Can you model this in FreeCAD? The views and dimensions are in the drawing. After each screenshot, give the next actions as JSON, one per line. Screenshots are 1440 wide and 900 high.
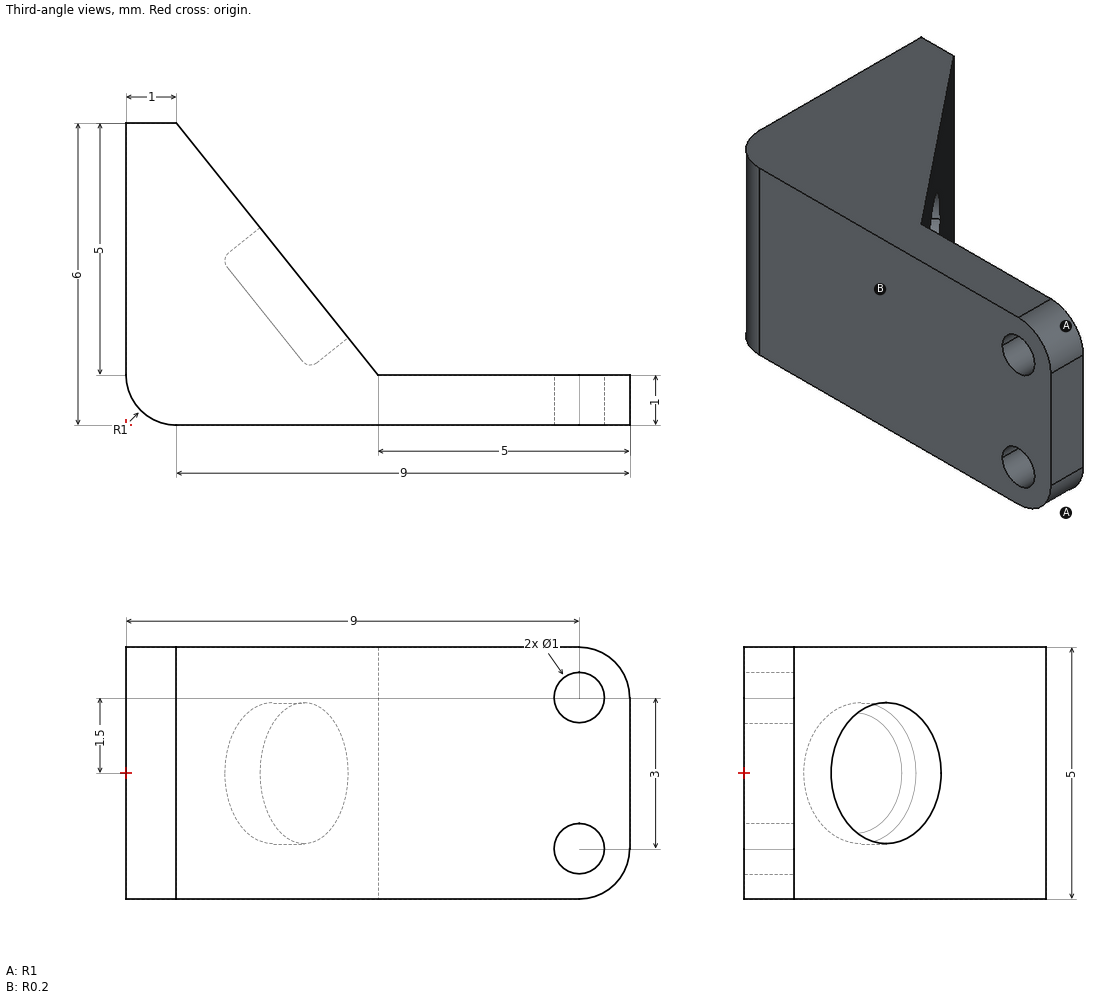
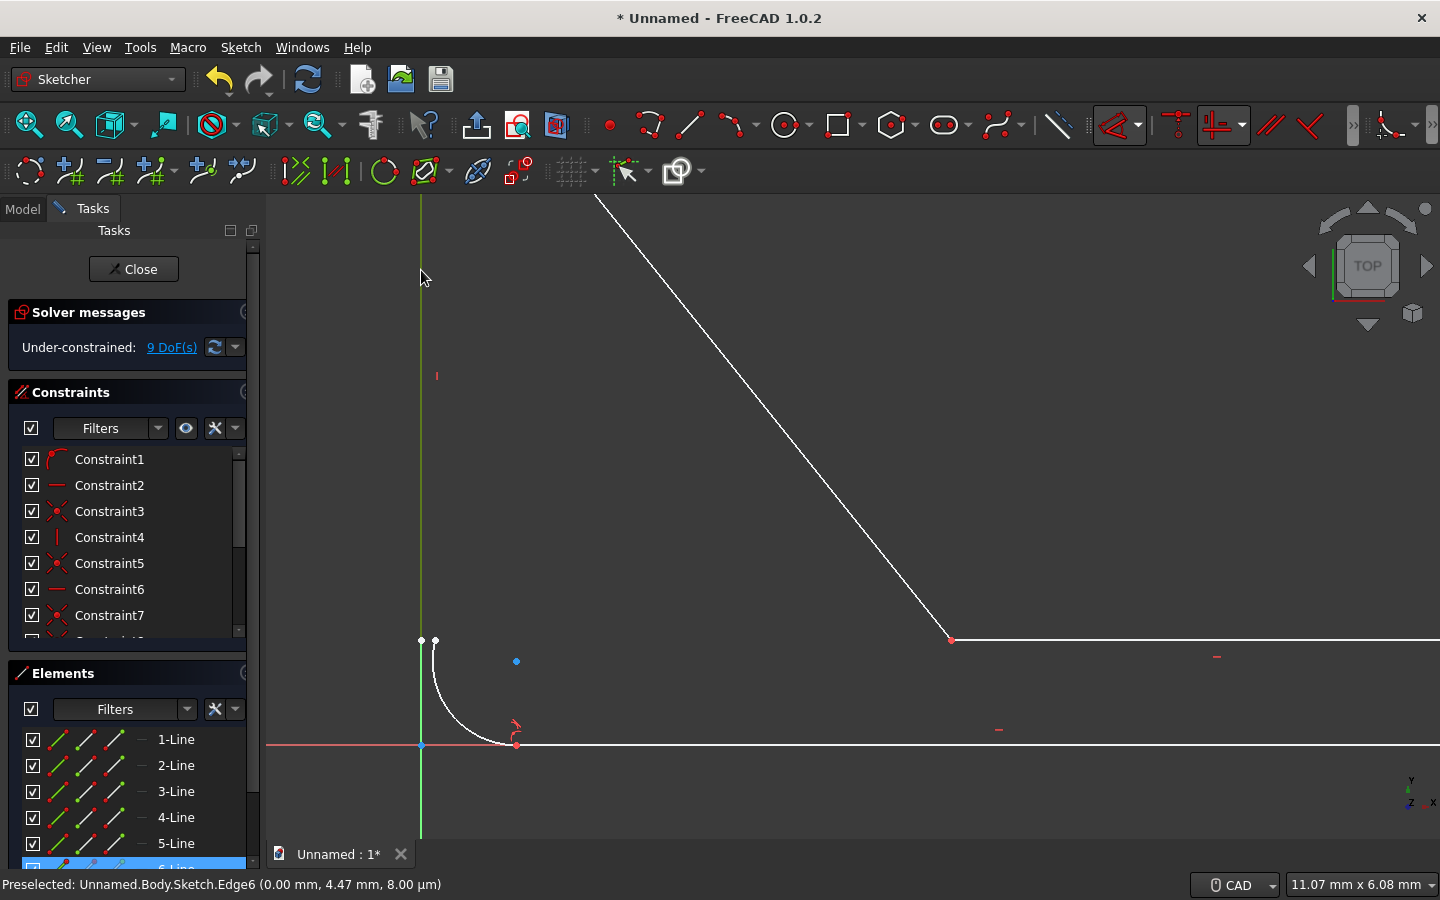
{"action": "left_click", "coordinate": [436, 686]}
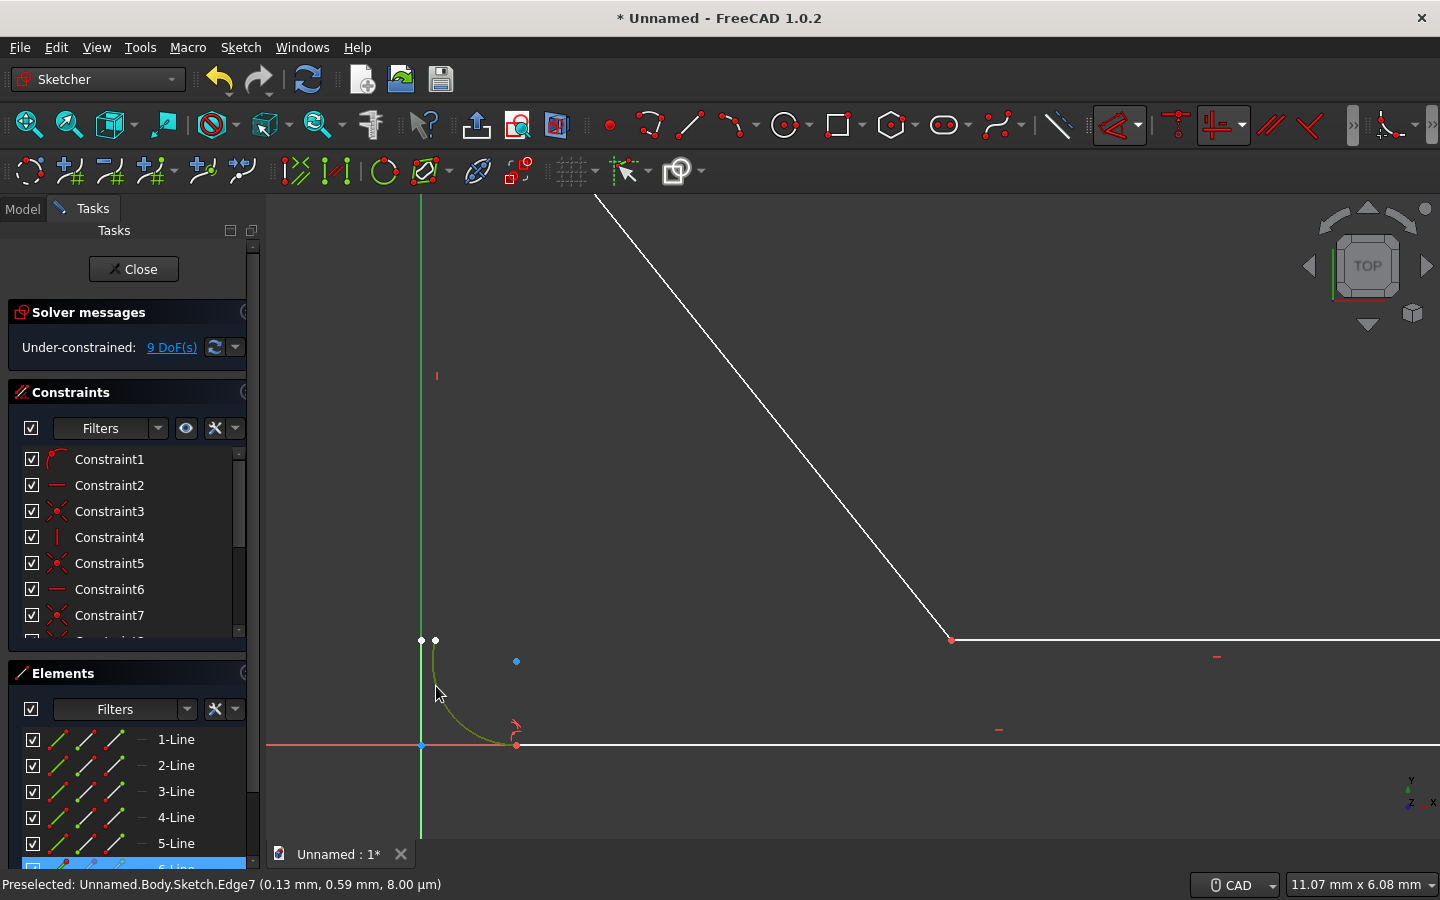
{"action": "key", "text": "t"}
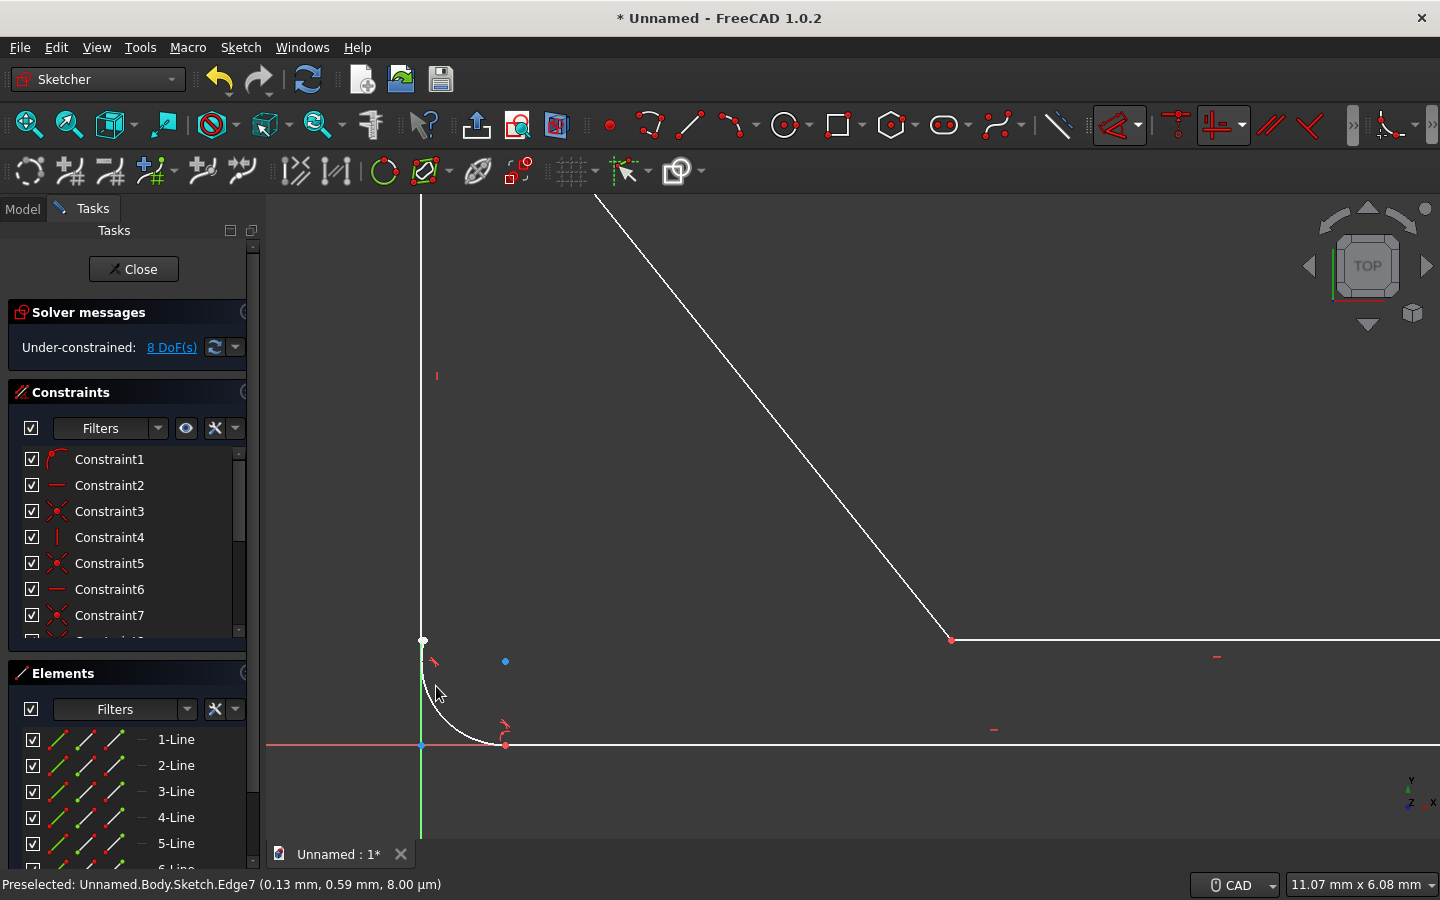
{"action": "left_click", "coordinate": [1114, 126]}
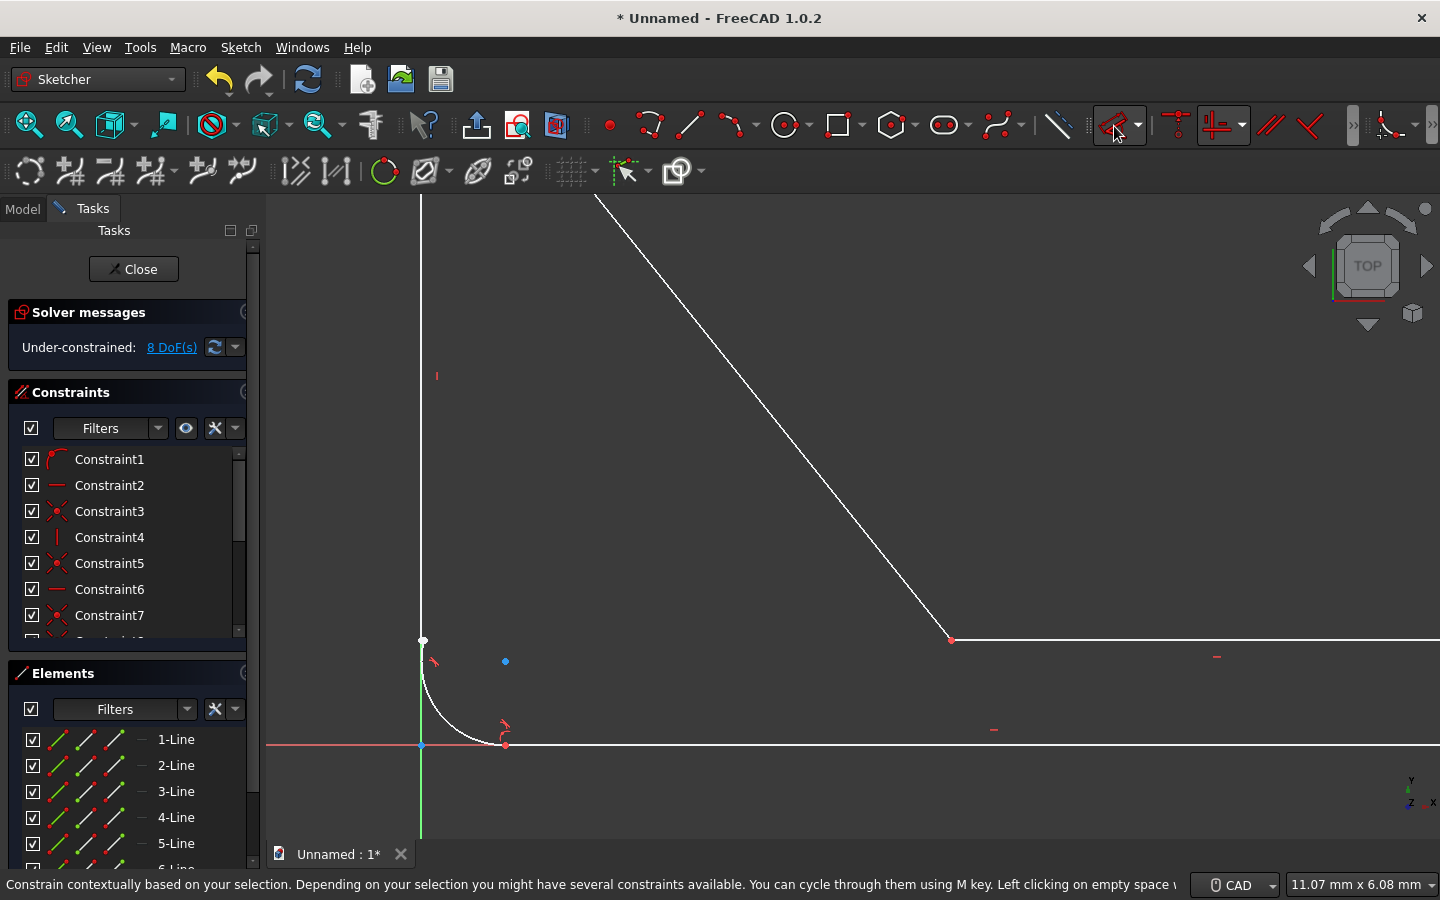
{"action": "left_click", "coordinate": [425, 686]}
{"action": "left_click", "coordinate": [394, 695]}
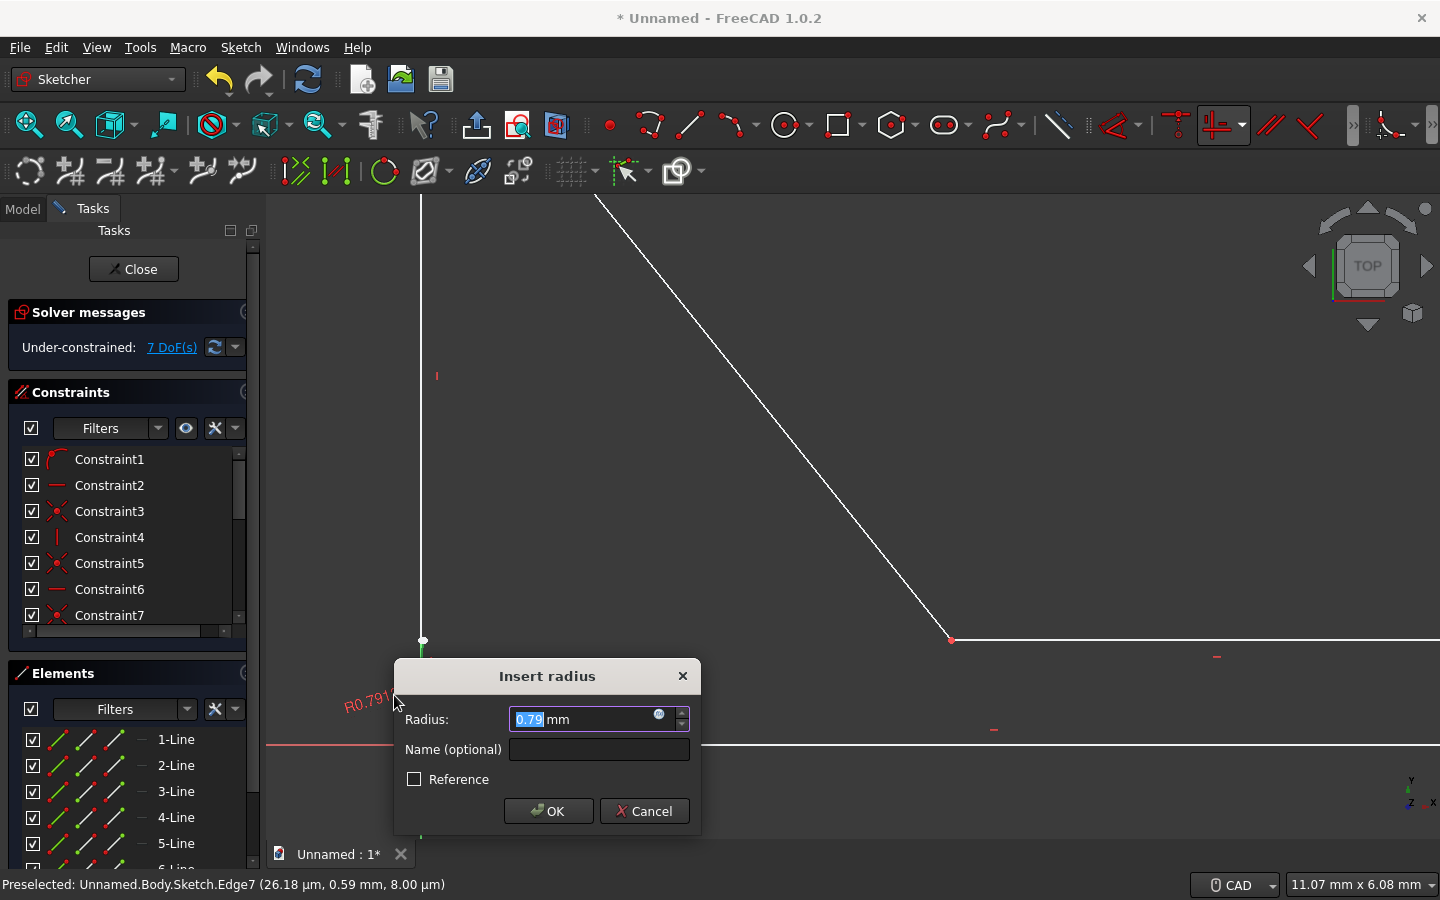
{"action": "type", "text": "1"}
{"action": "key", "text": "Return"}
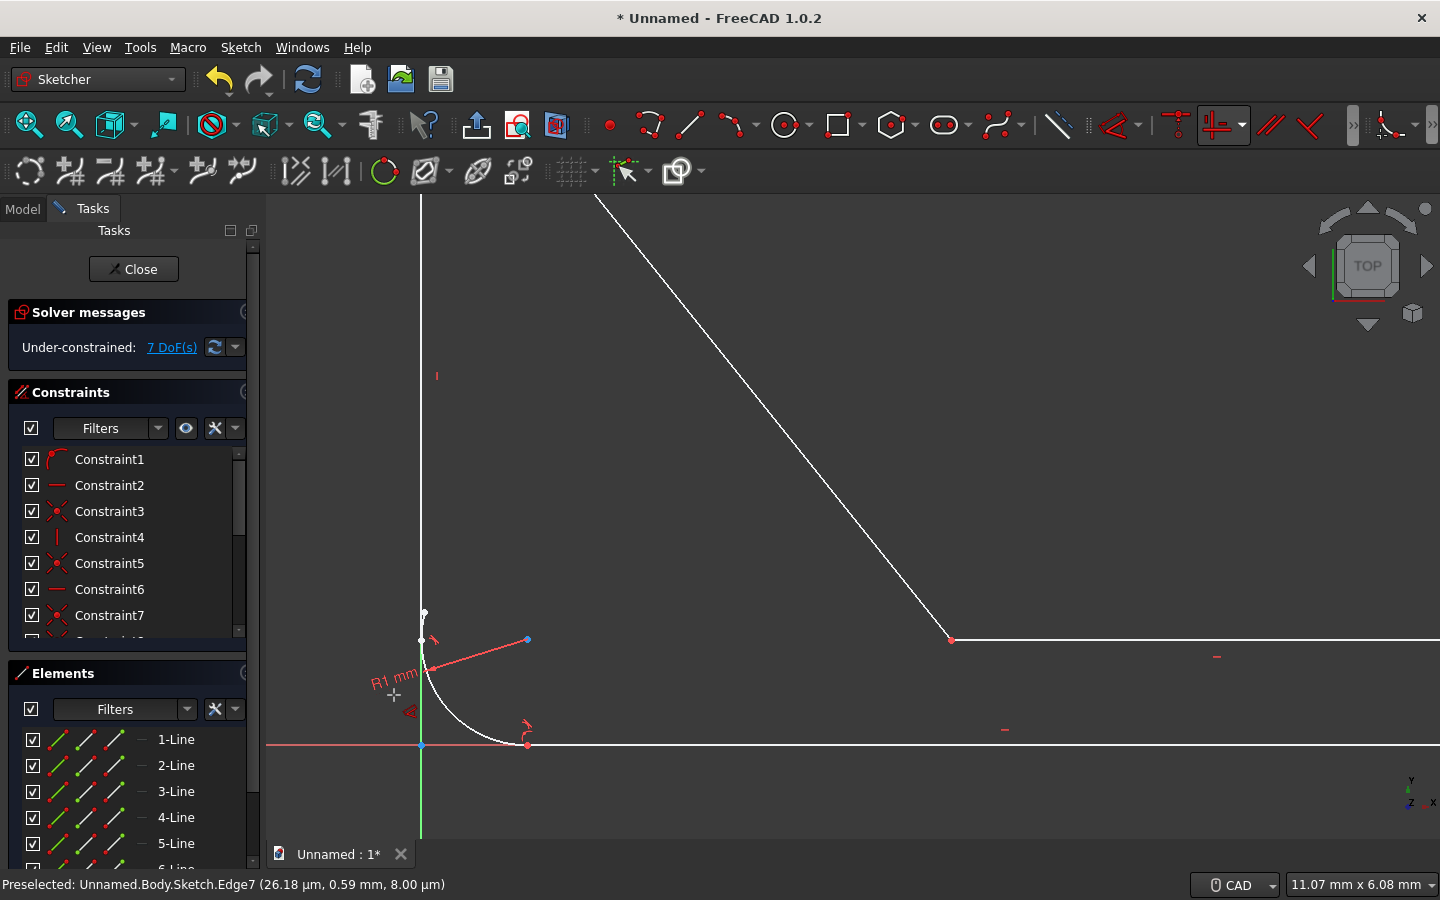
{"action": "left_click", "coordinate": [814, 745]}
{"action": "left_click", "coordinate": [901, 779]}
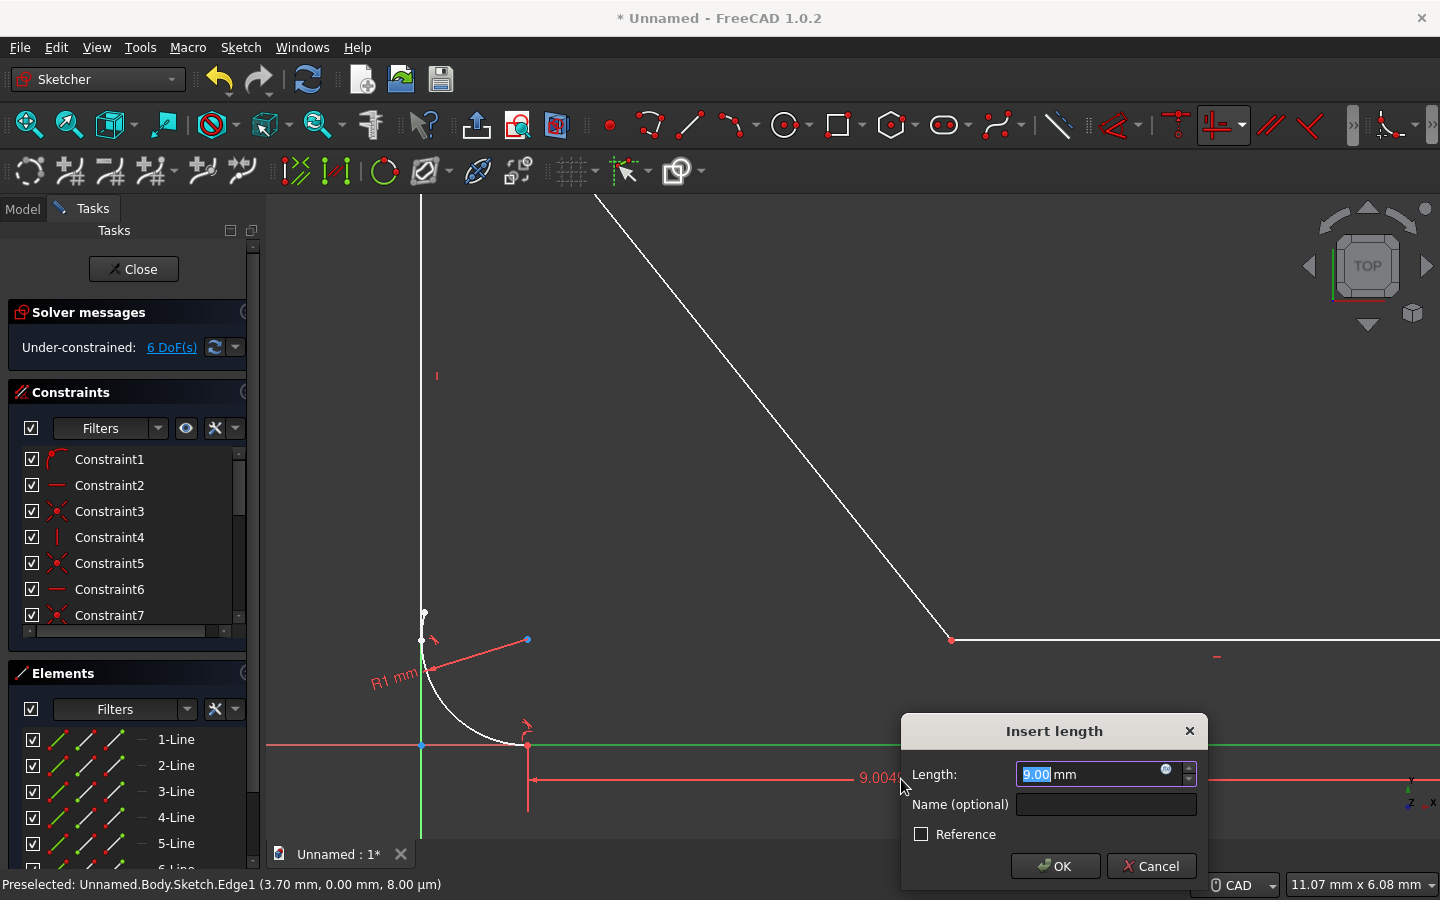
{"action": "type", "text": "9"}
{"action": "key", "text": "Return"}